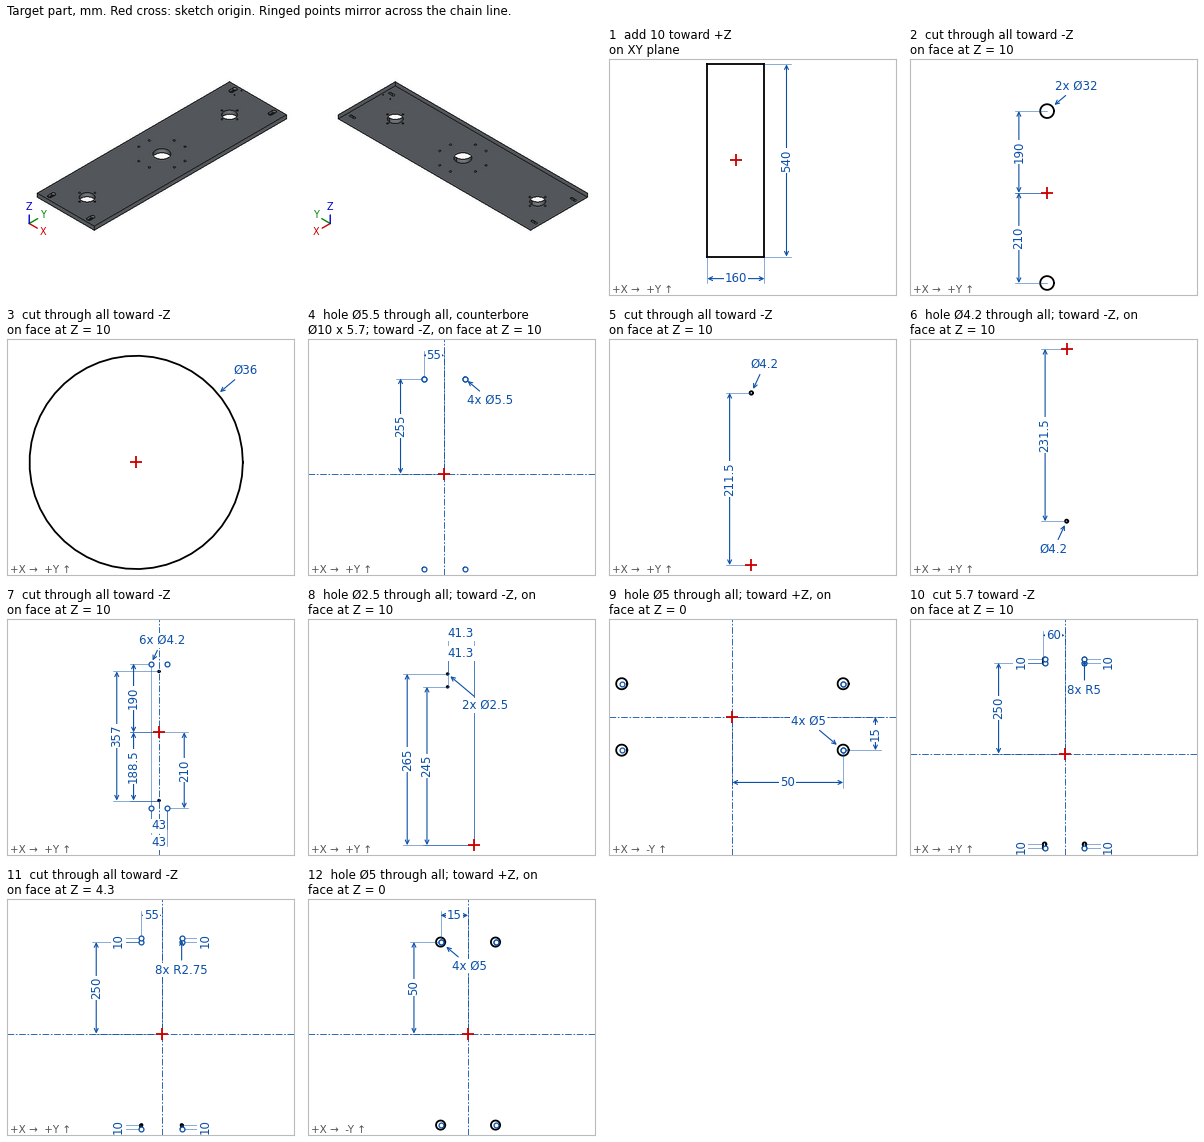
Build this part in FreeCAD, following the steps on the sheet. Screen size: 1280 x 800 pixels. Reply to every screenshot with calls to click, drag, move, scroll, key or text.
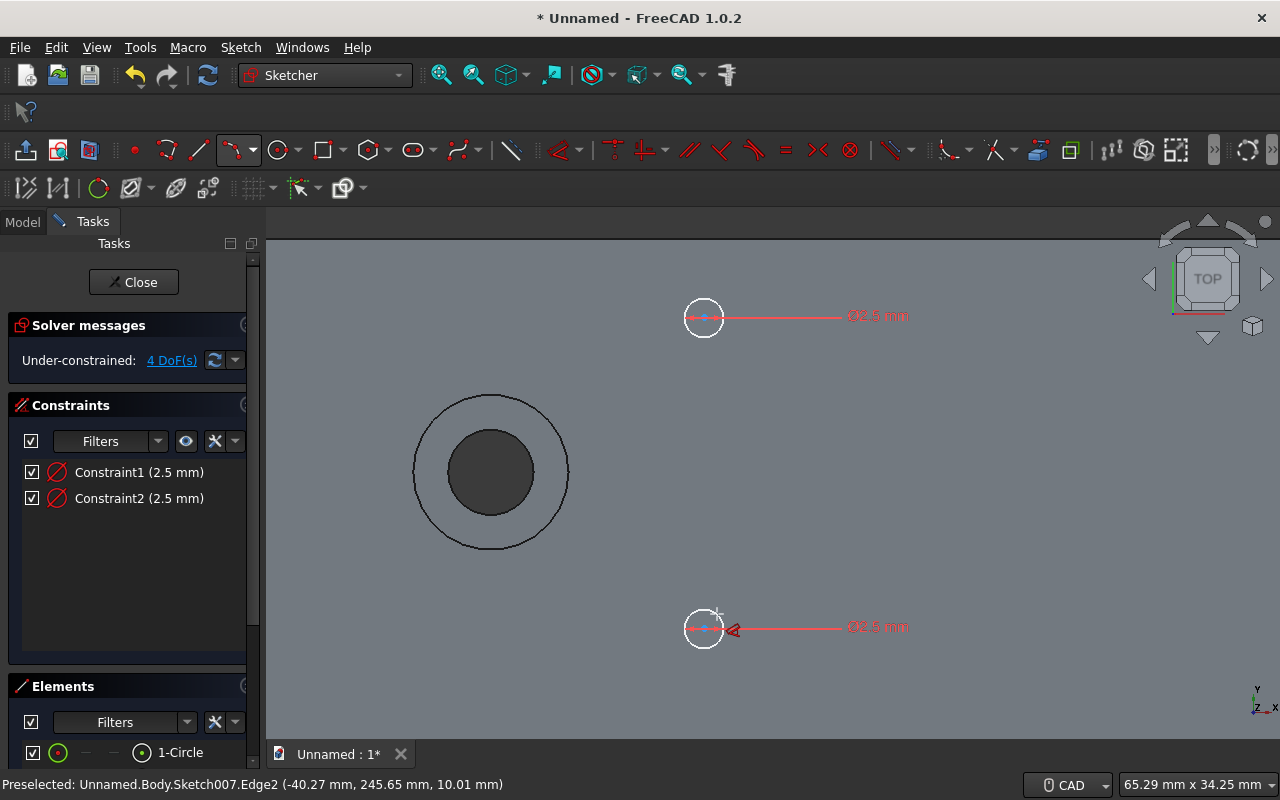
click(704, 318)
click(670, 514)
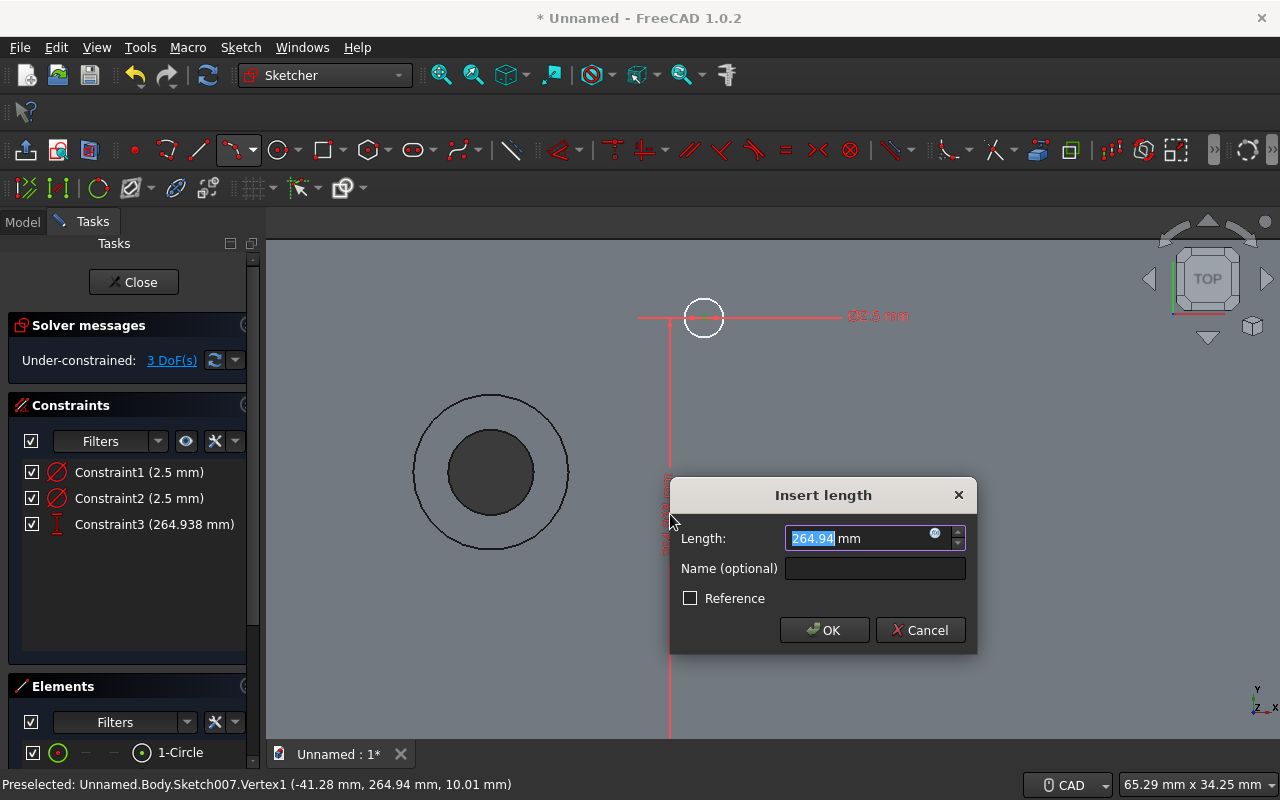
text(265)
key(Return)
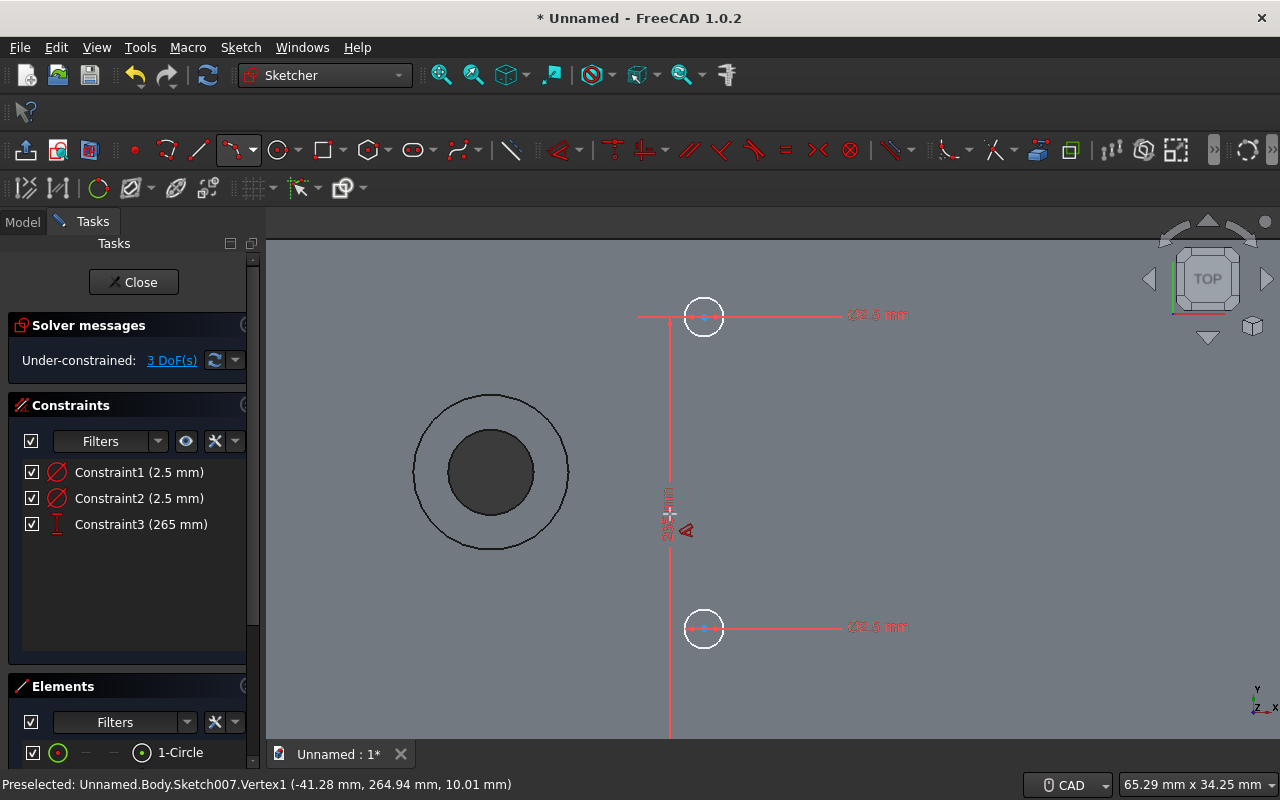
click(704, 629)
click(670, 670)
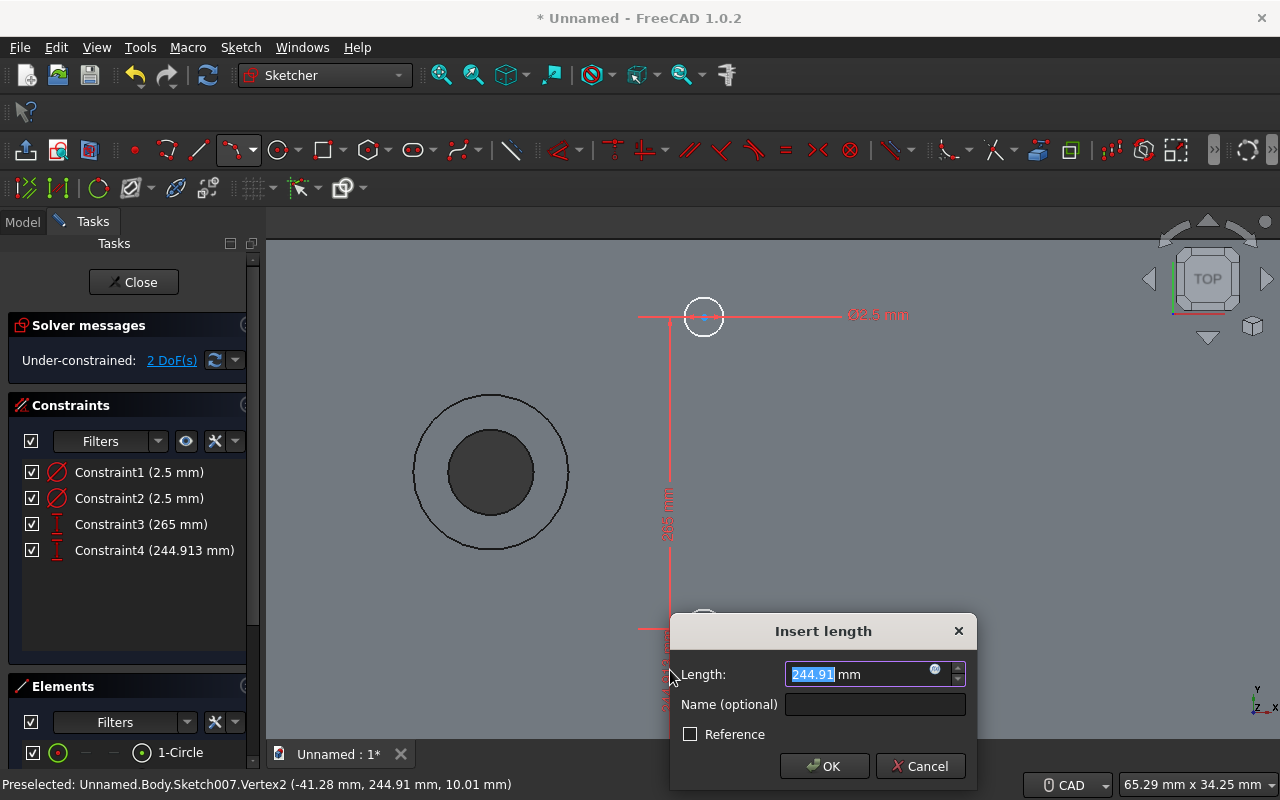
text(245)
key(Return)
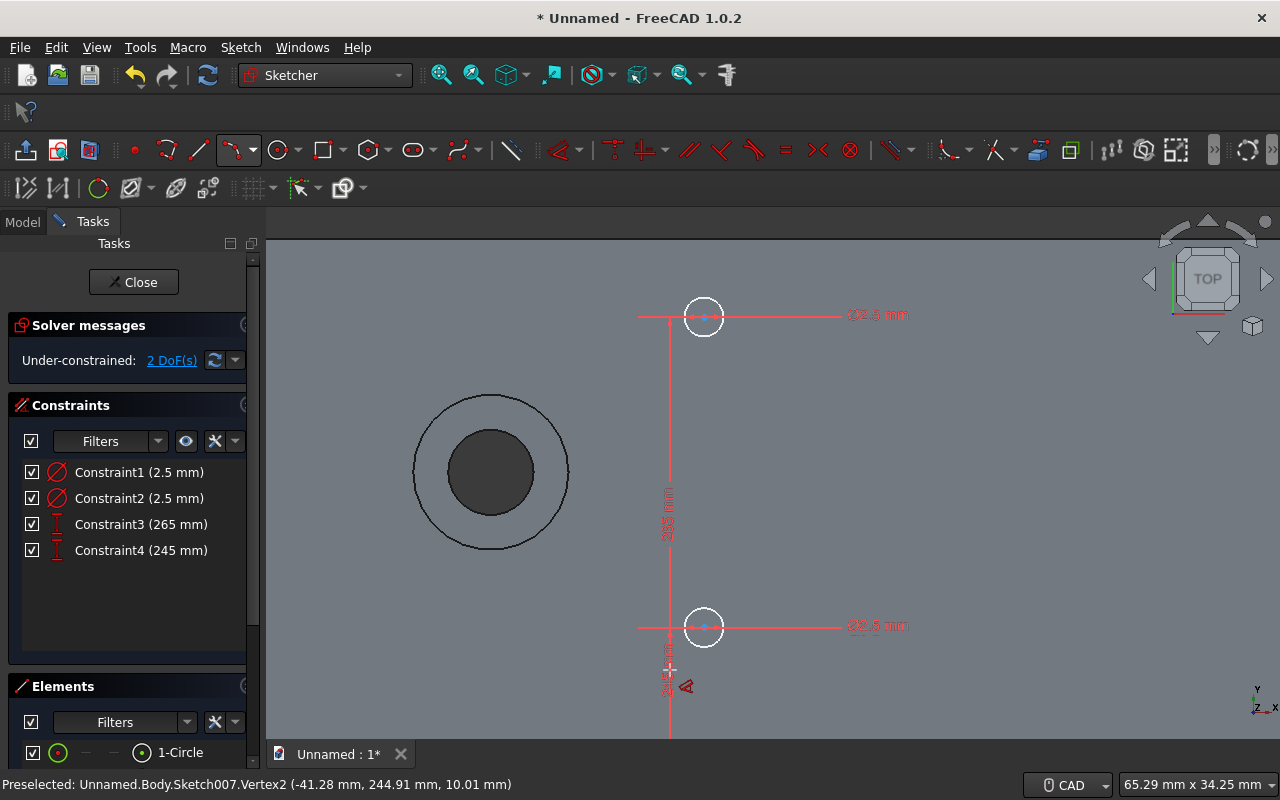
click(704, 317)
click(910, 283)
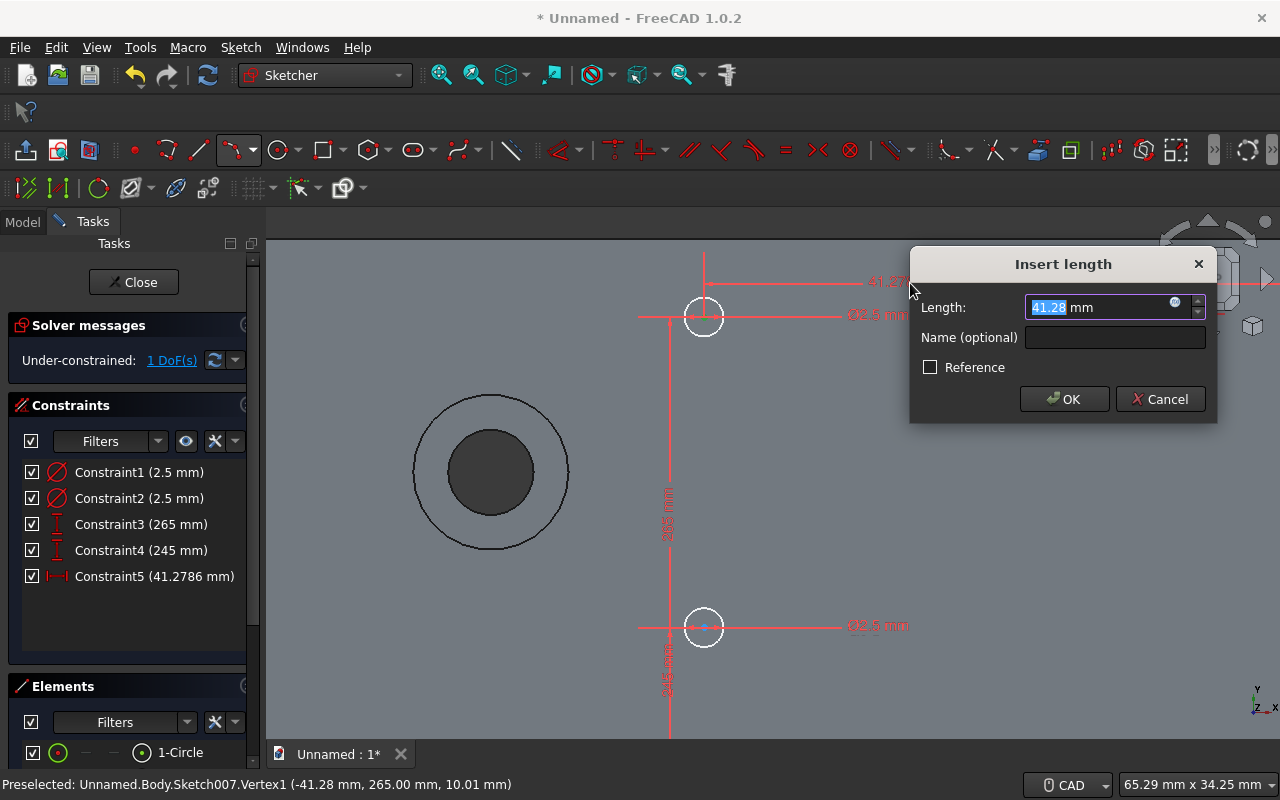
text(41.3)
key(Return)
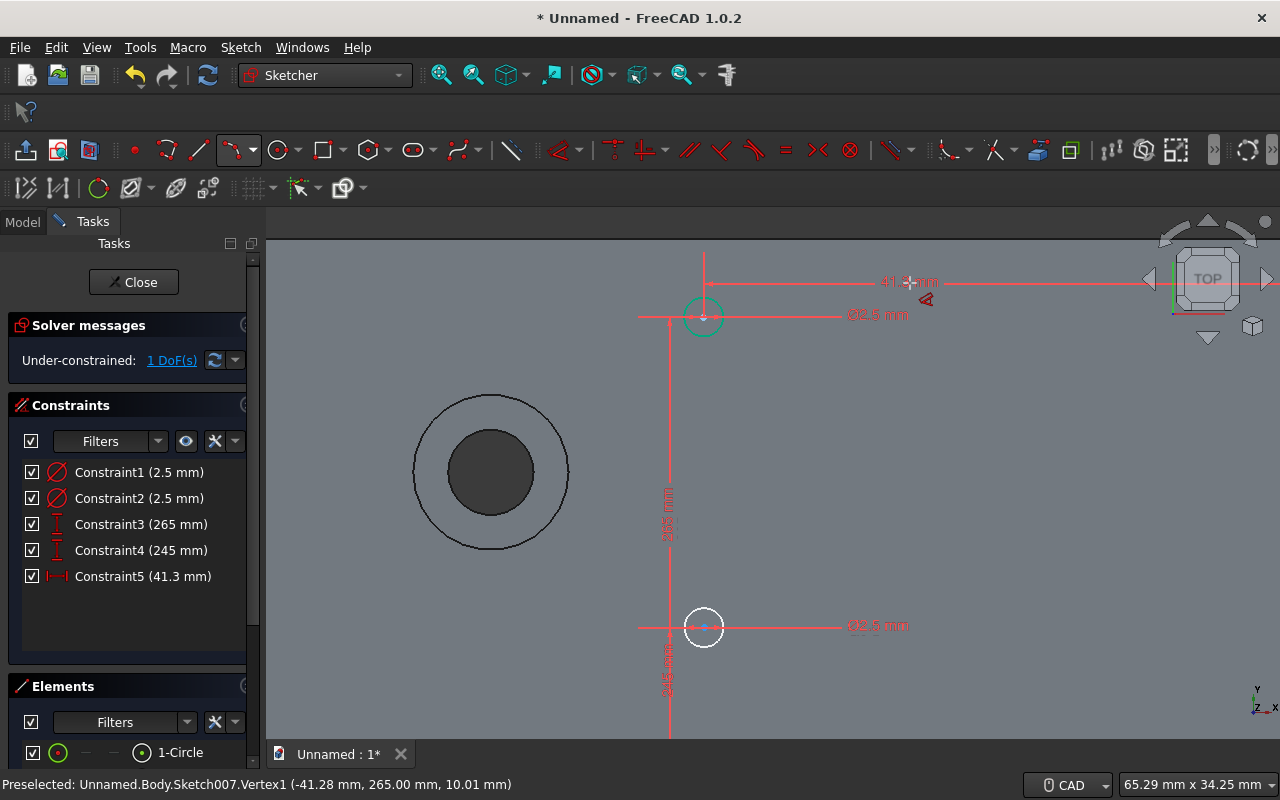
click(704, 628)
click(910, 594)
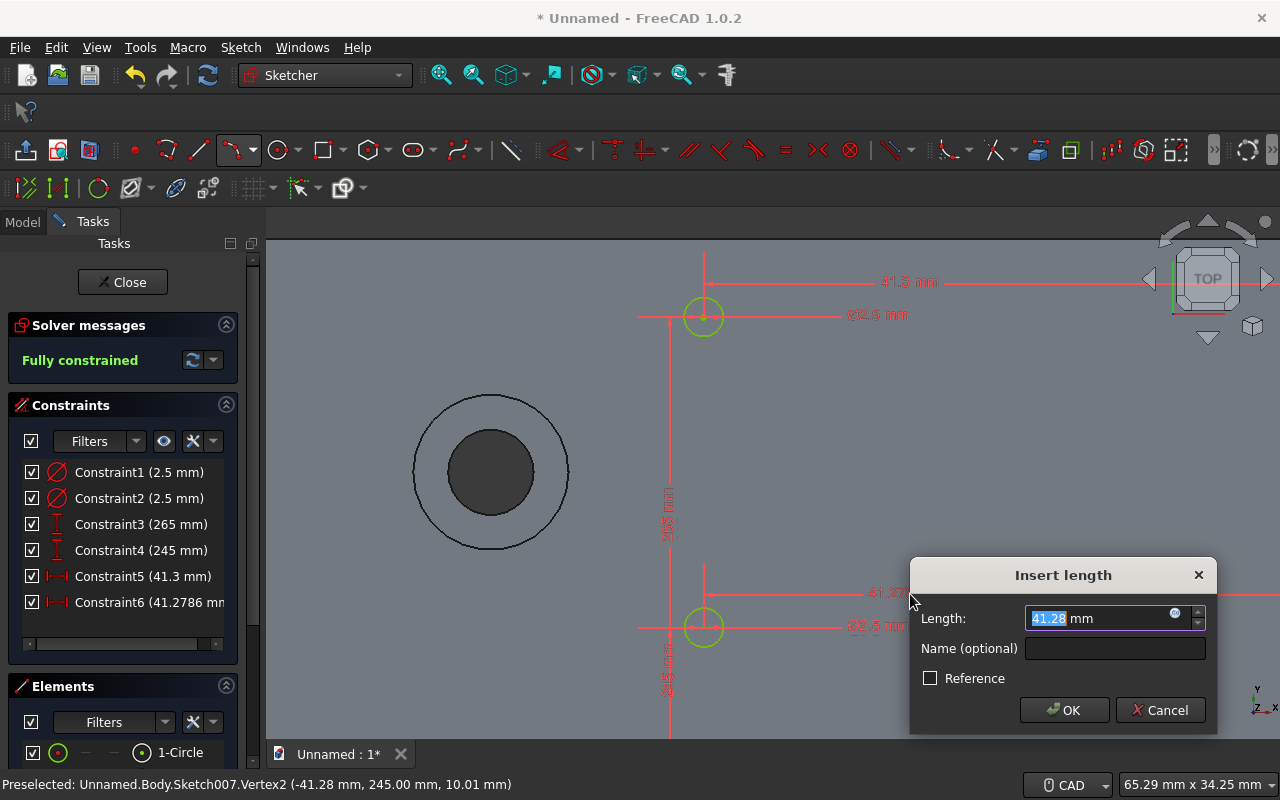
text(41.3)
key(Return)
key(Escape)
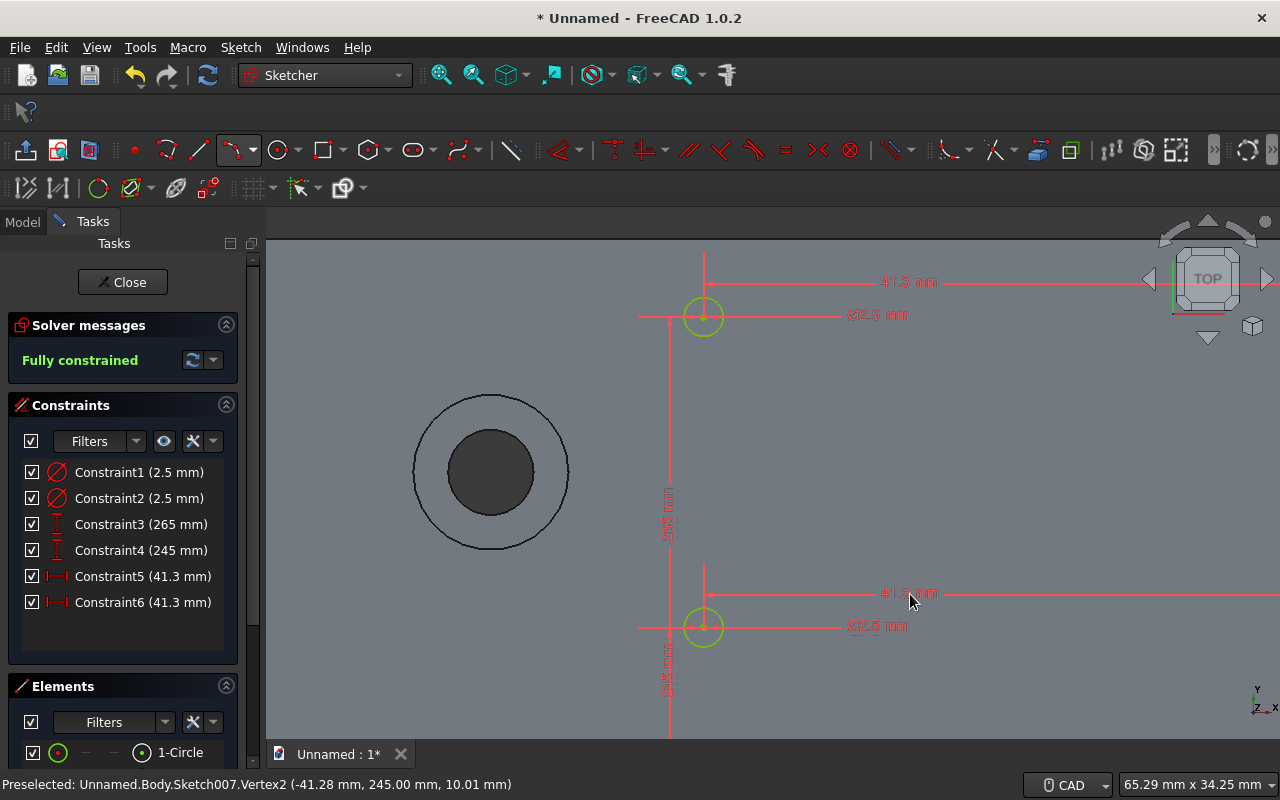
click(123, 282)